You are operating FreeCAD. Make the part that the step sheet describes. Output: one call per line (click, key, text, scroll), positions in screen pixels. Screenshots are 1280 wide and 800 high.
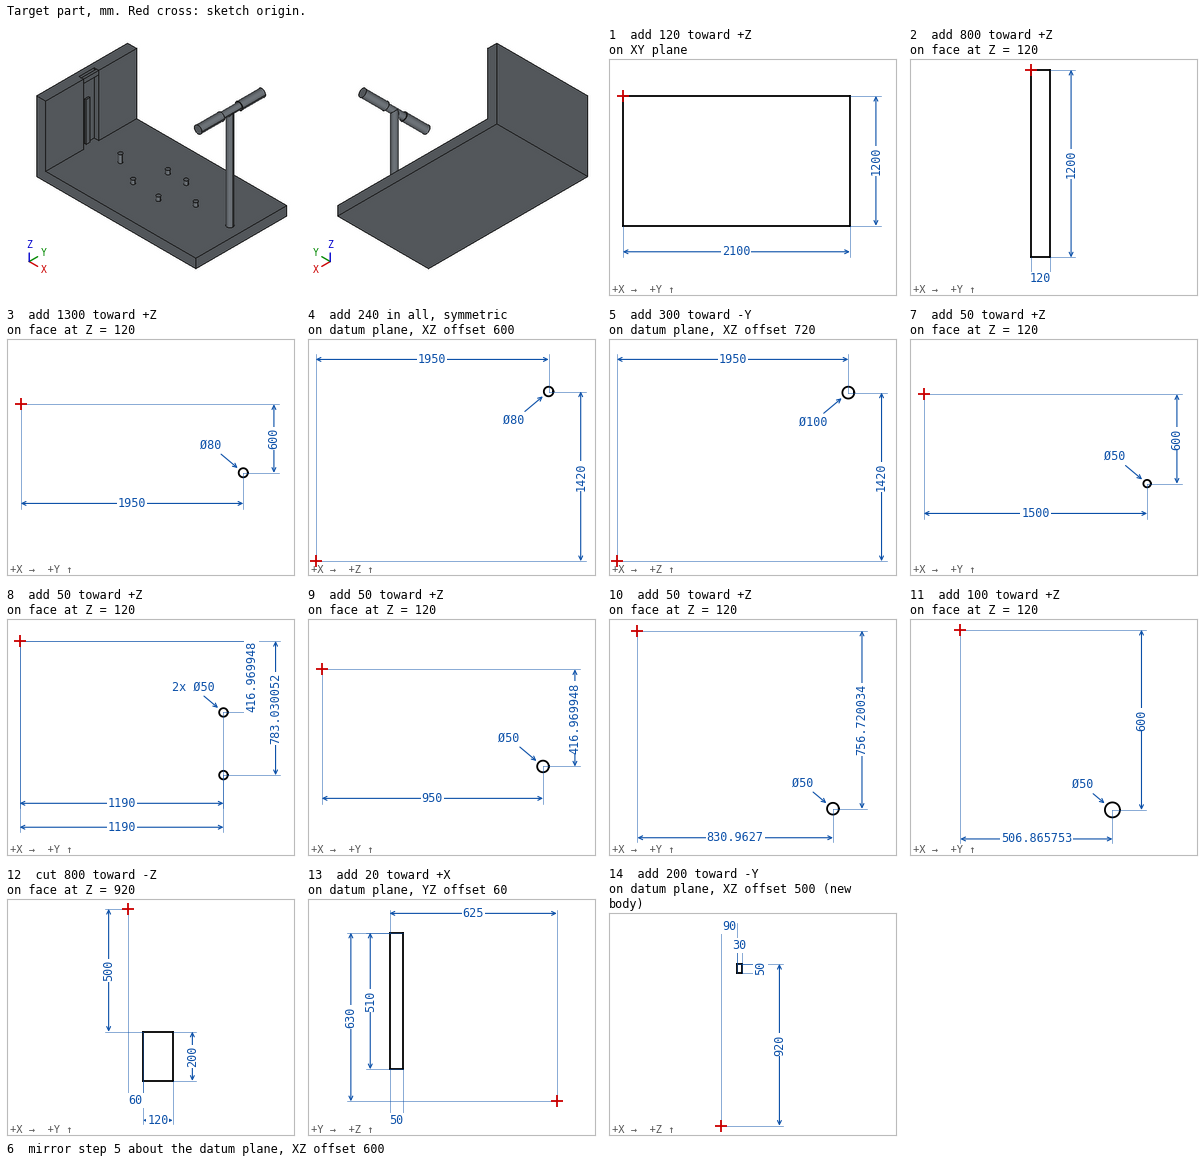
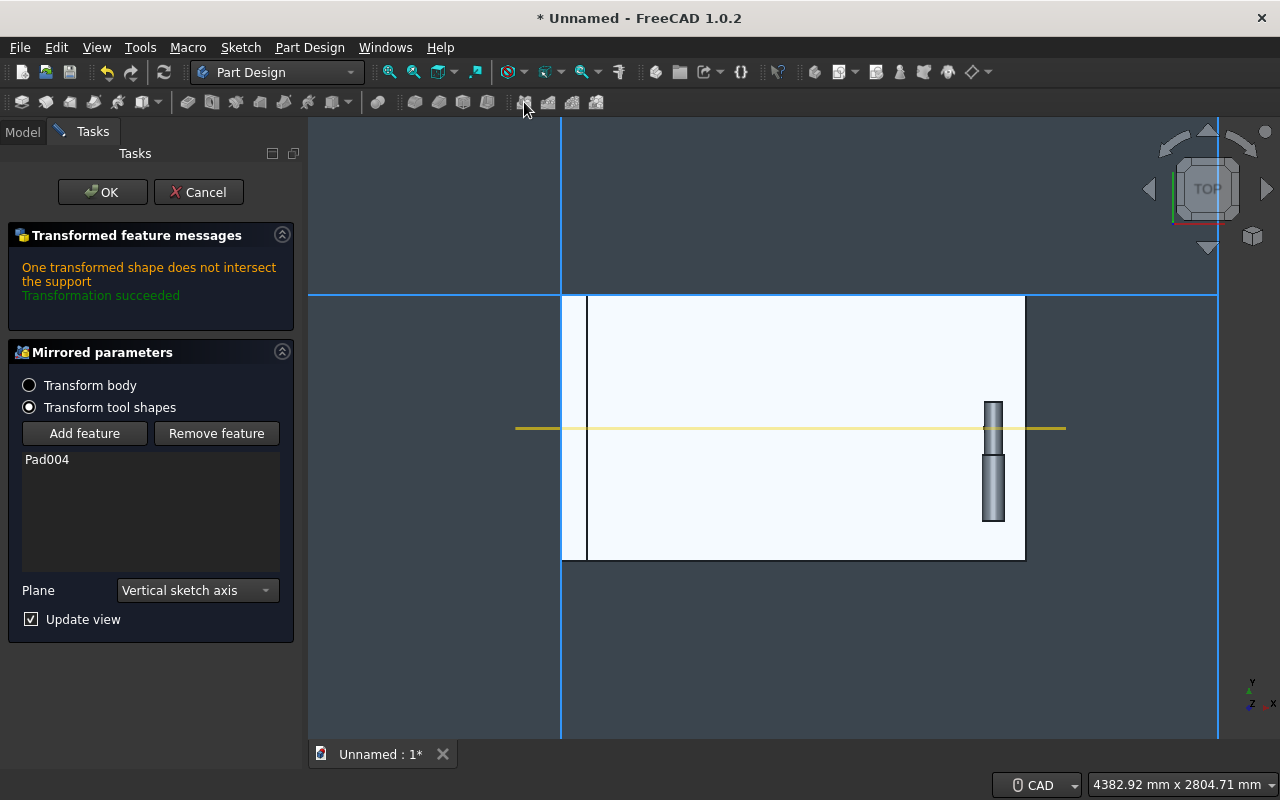
click(198, 590)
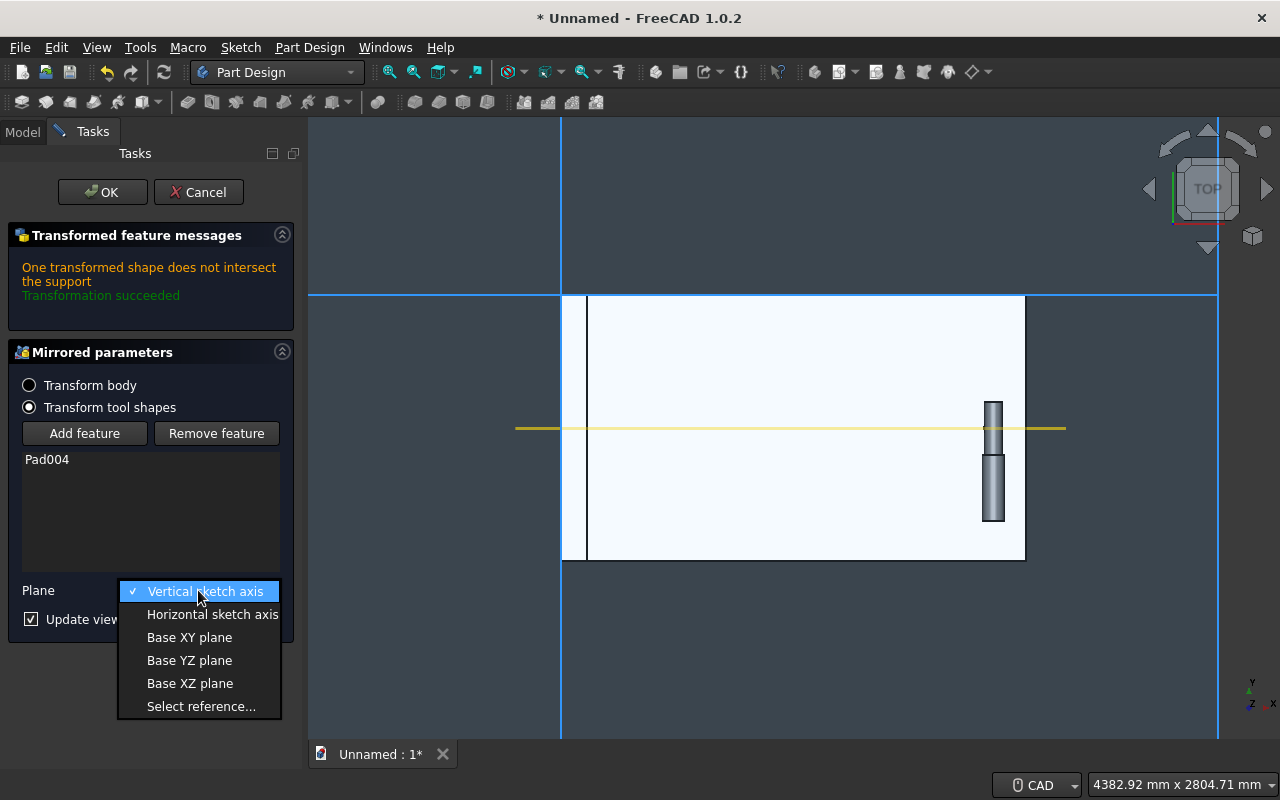
click(198, 706)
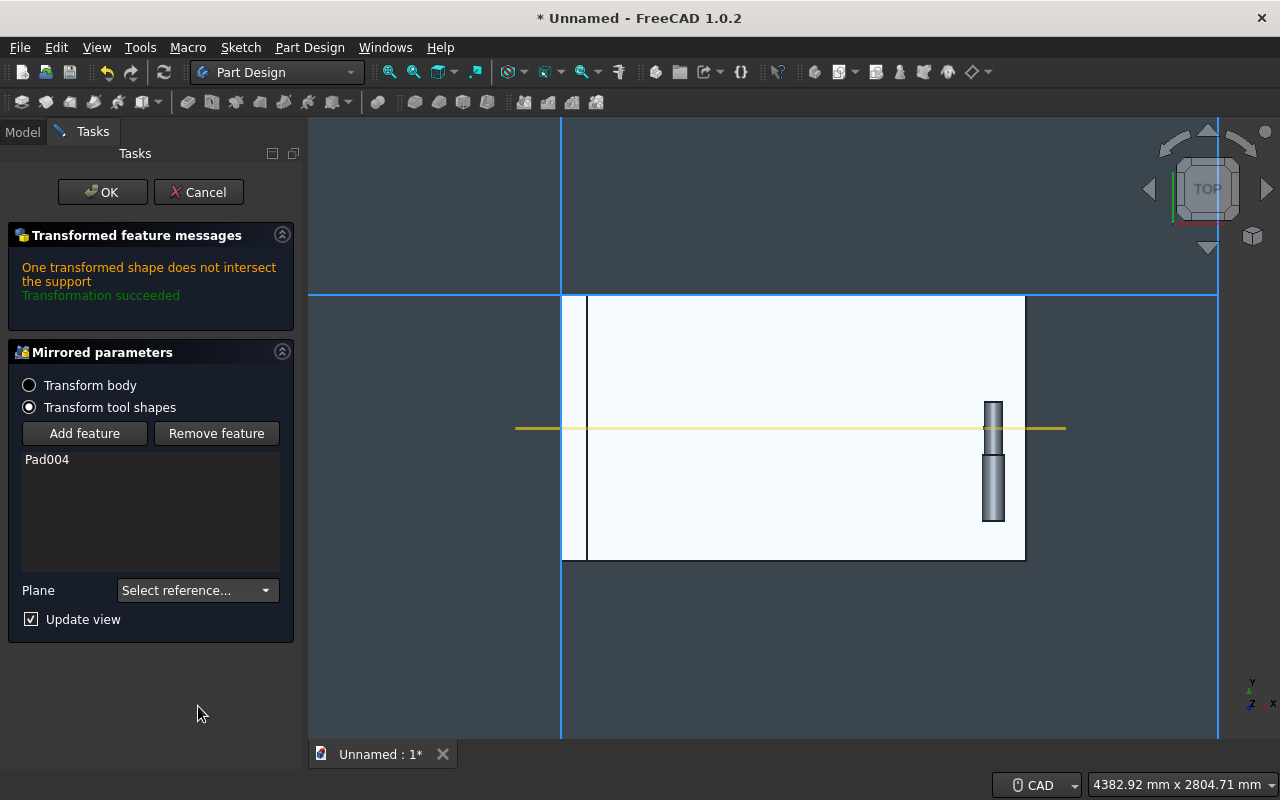
click(23, 131)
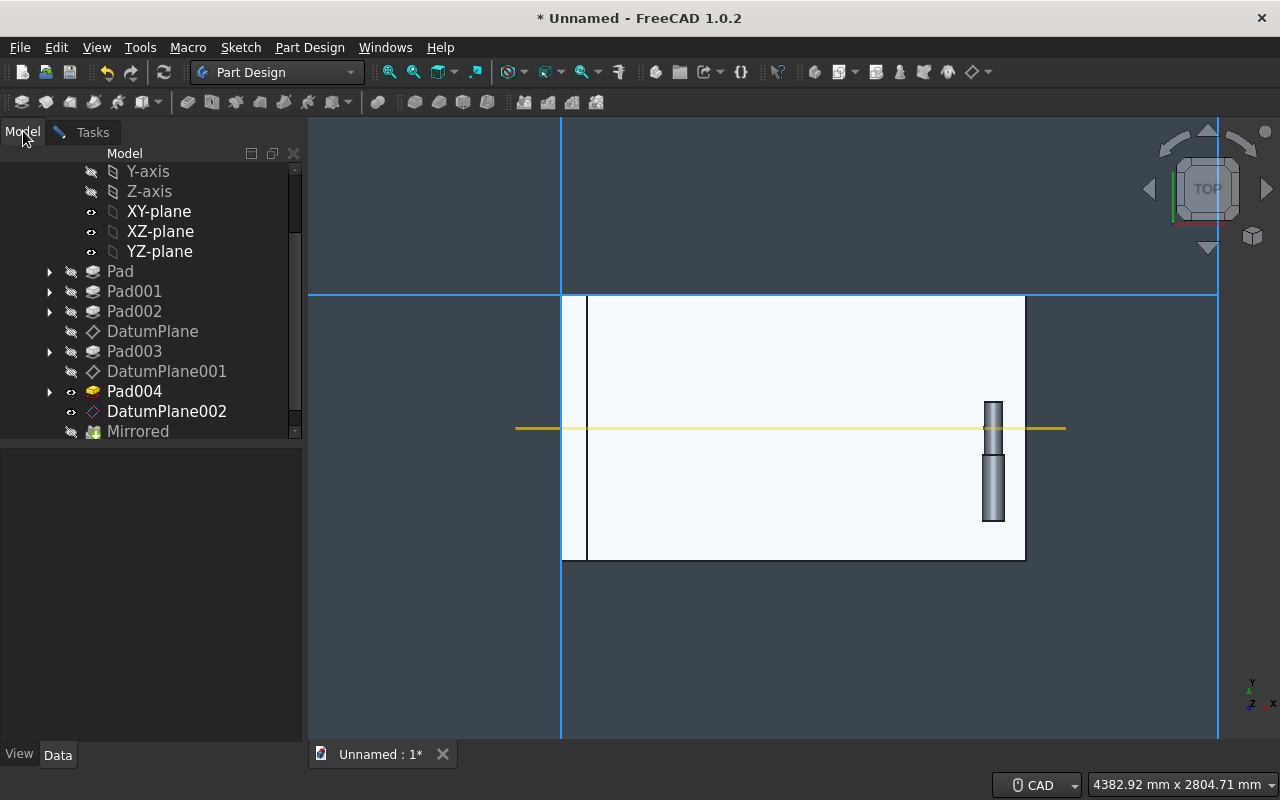
click(116, 412)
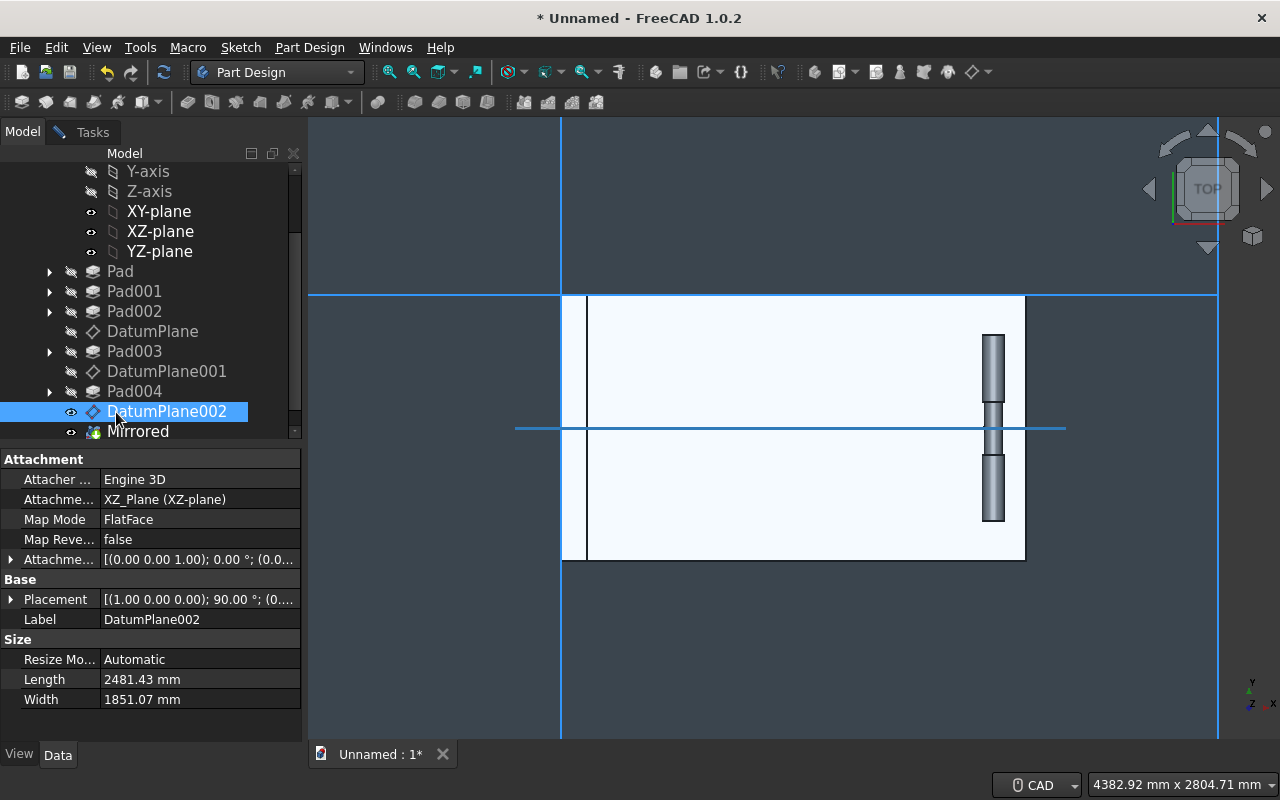
click(84, 131)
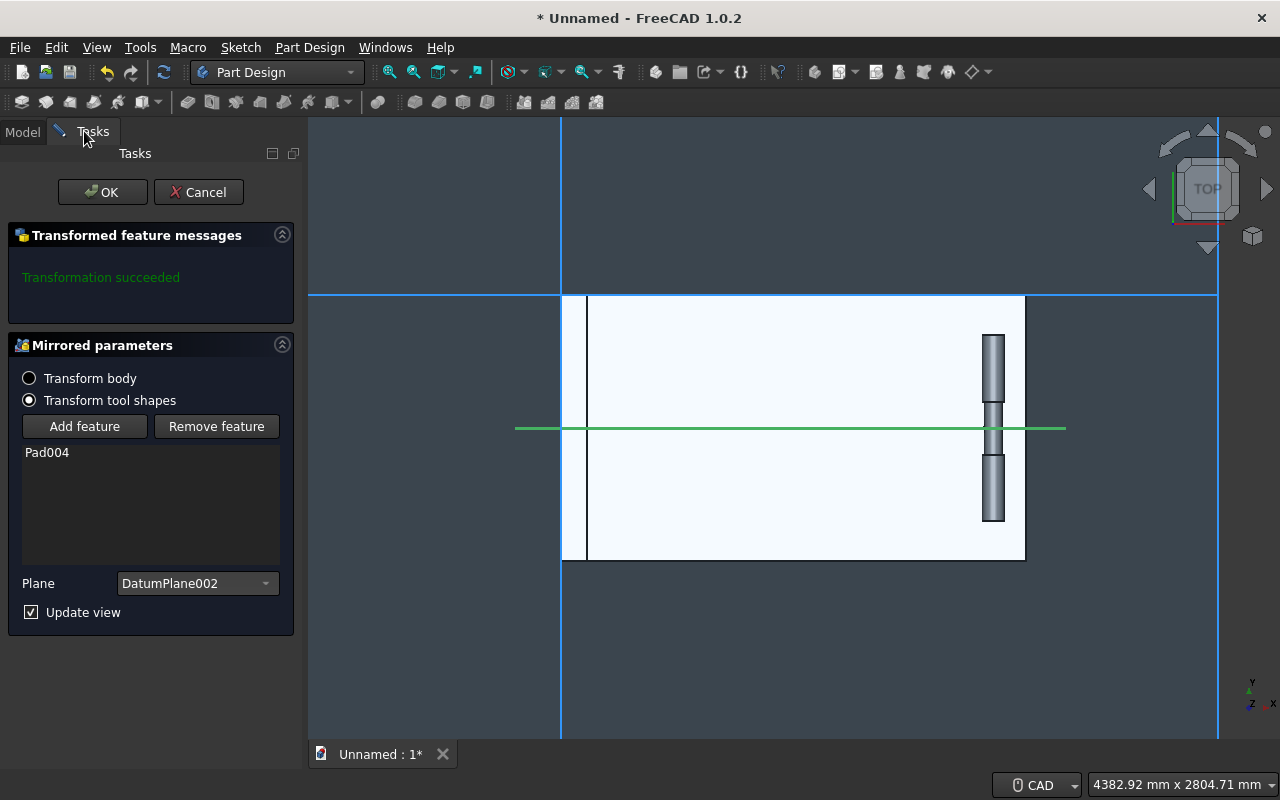
click(103, 192)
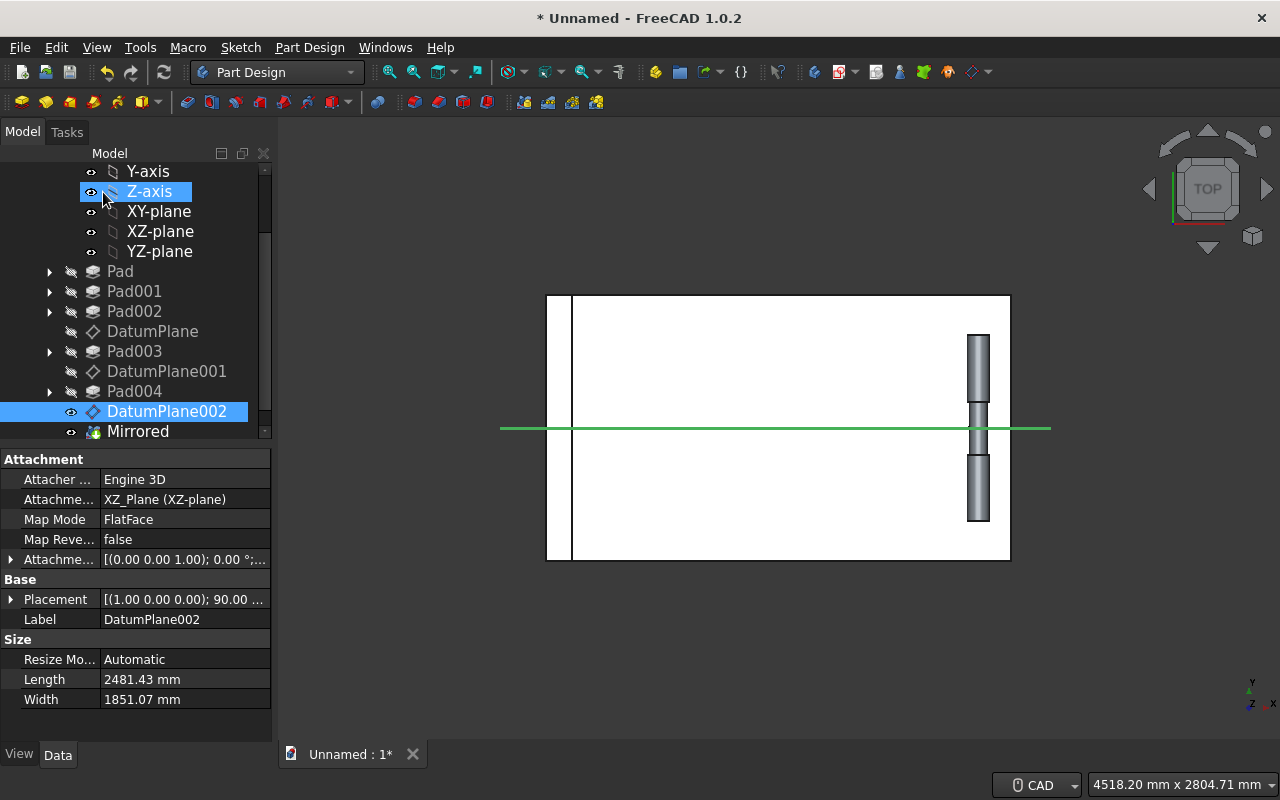
click(116, 412)
key(space)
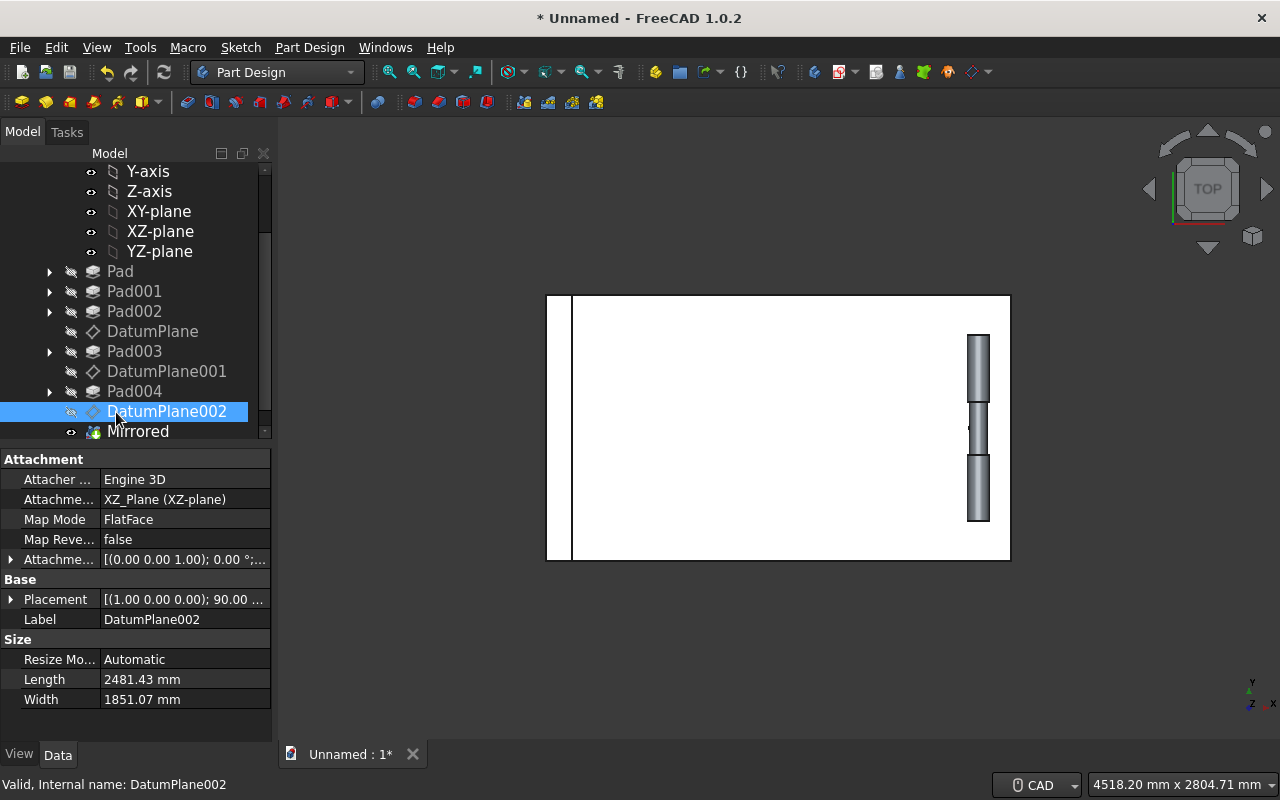
click(792, 427)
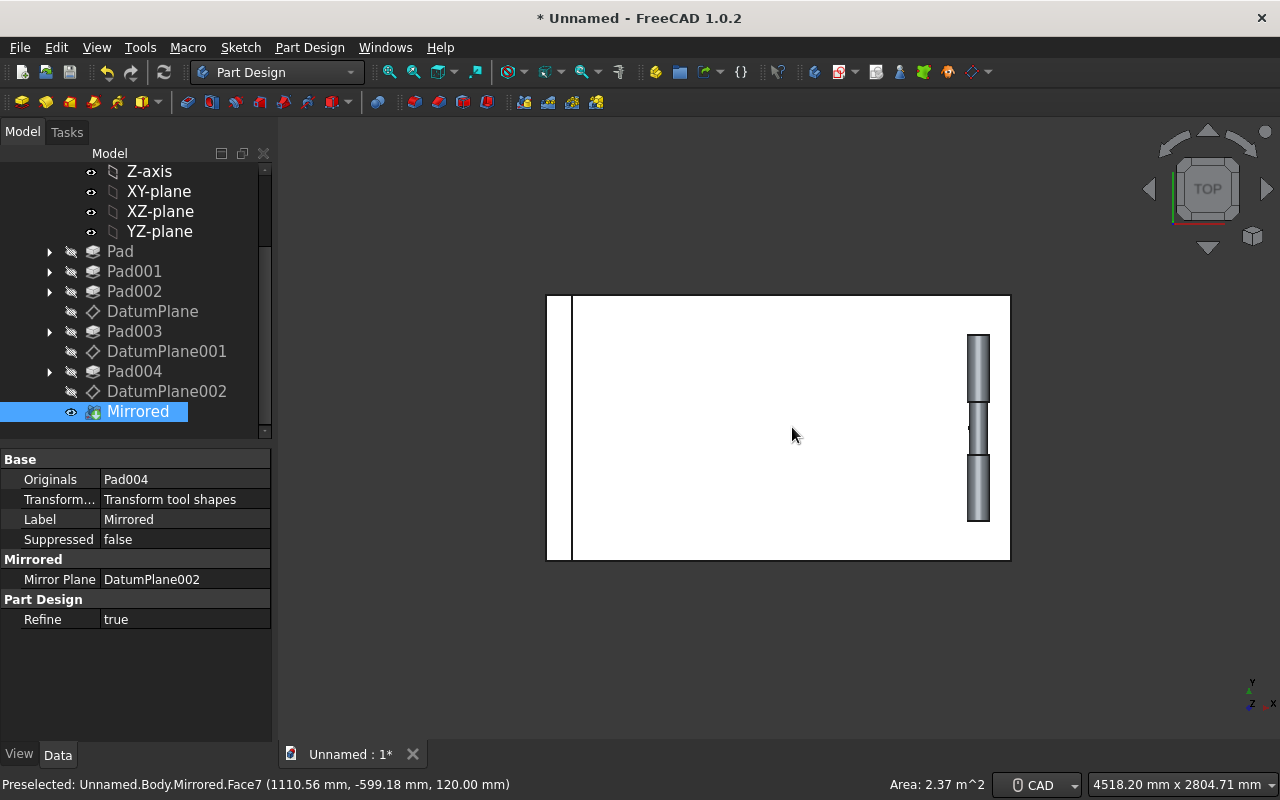
click(840, 72)